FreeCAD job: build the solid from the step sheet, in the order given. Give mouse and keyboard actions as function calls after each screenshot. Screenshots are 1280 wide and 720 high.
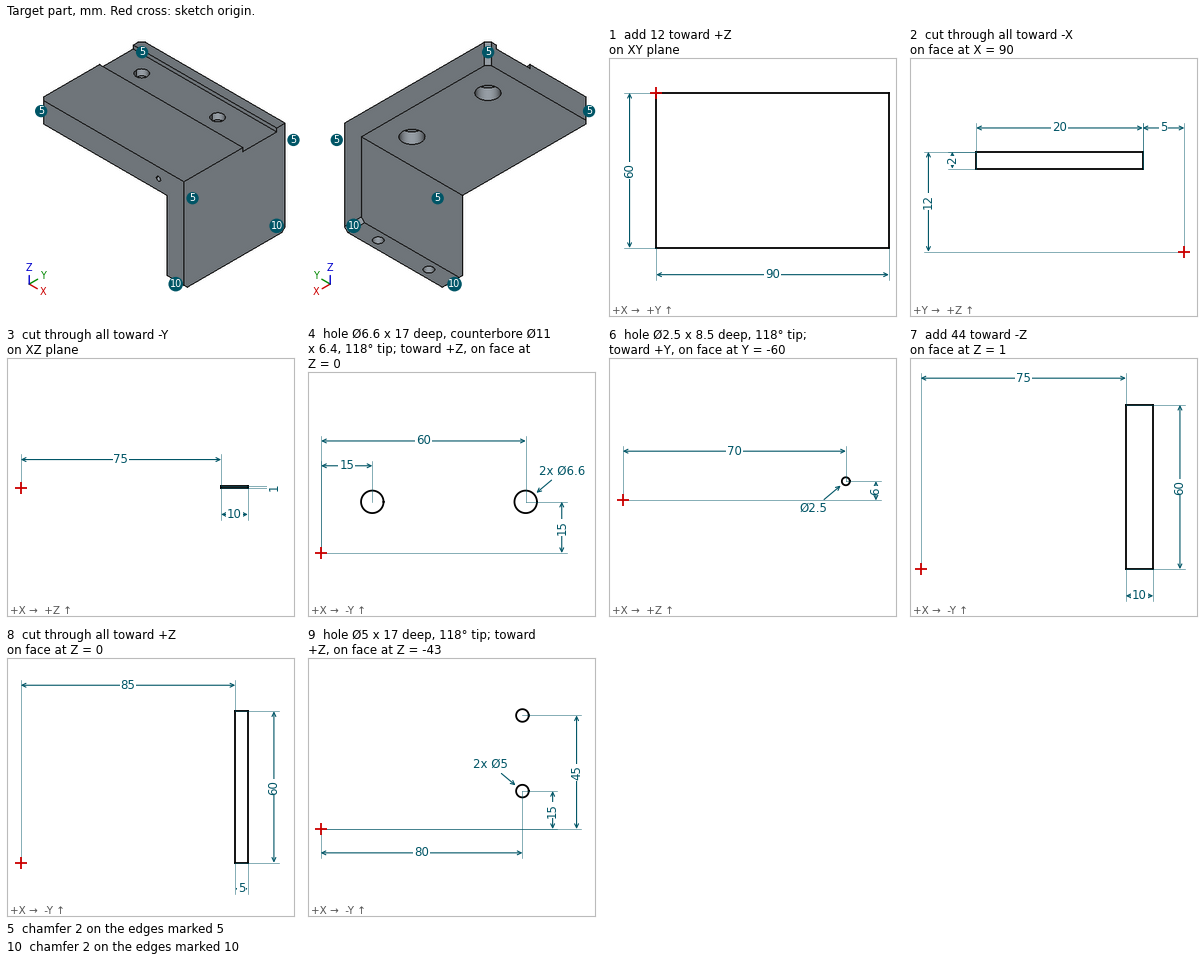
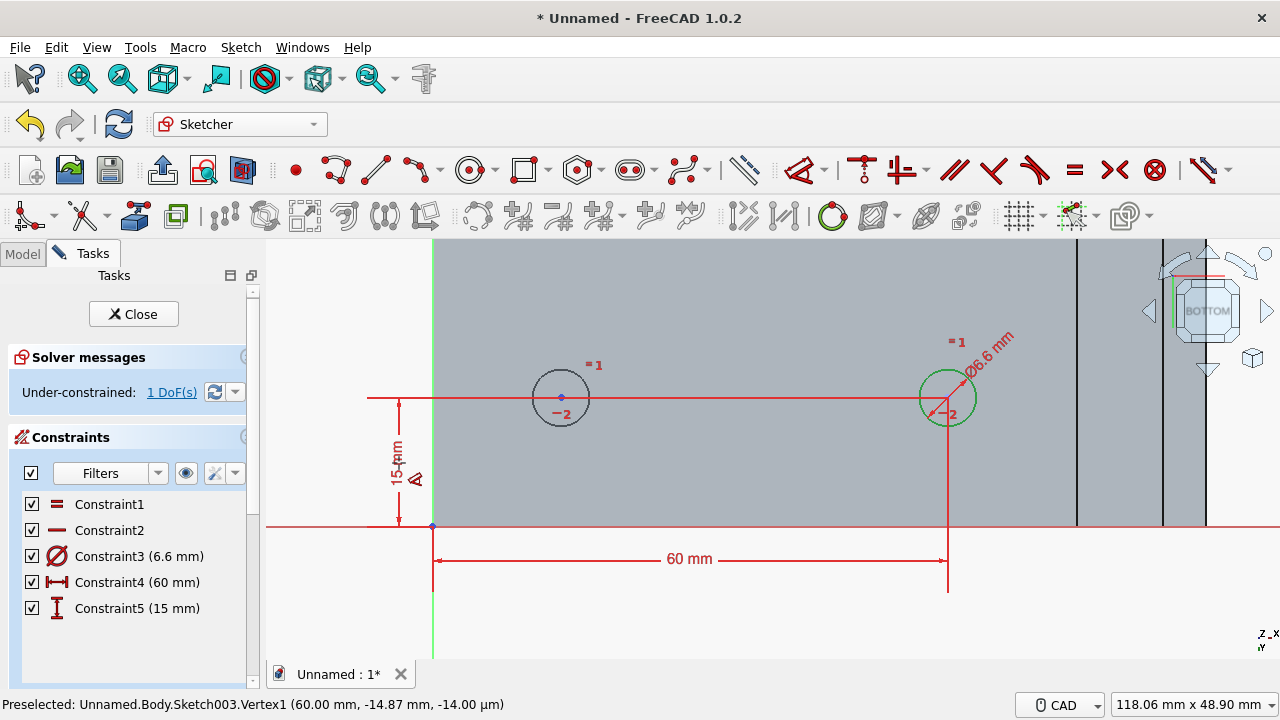
click(561, 398)
click(497, 561)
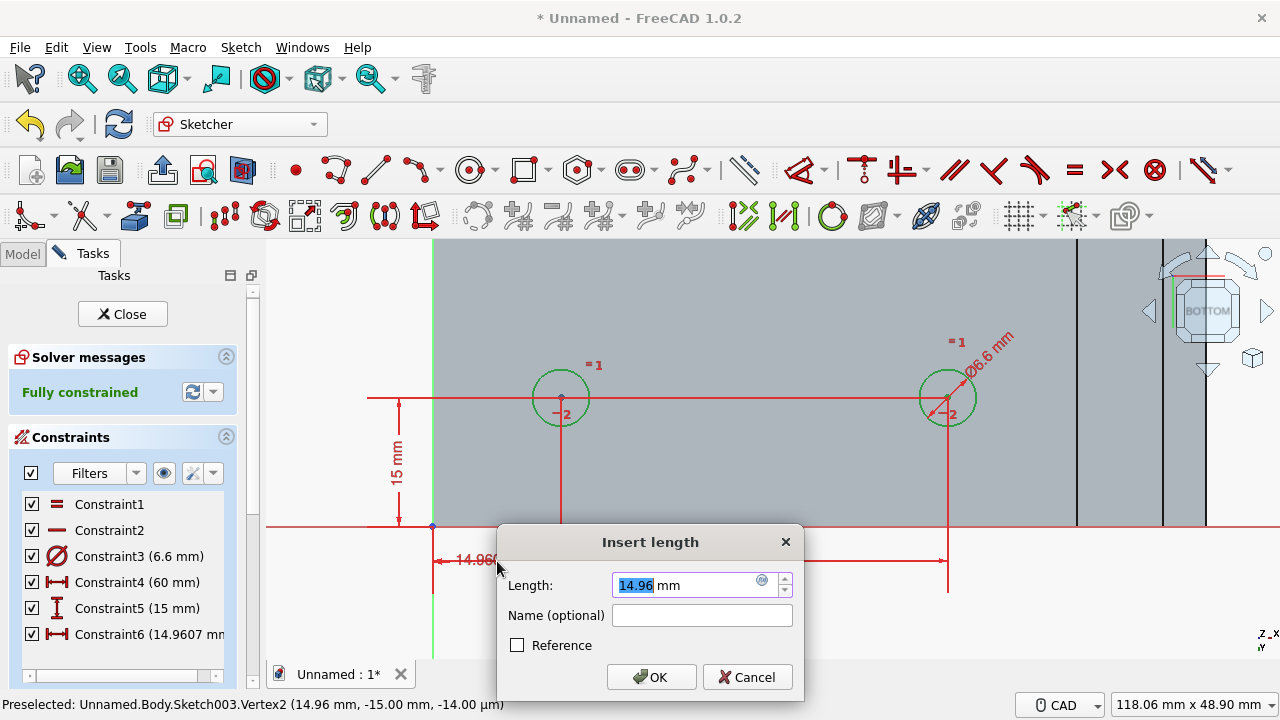
text(15)
key(Return)
key(Escape)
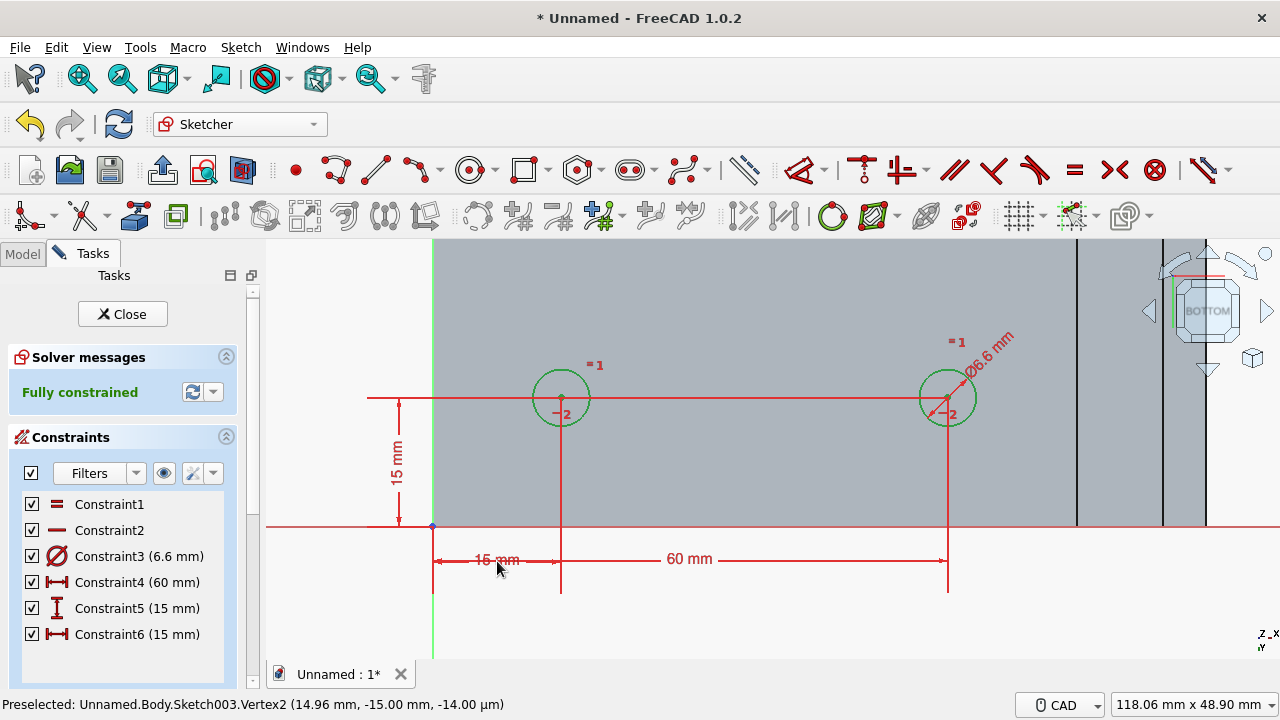
click(123, 314)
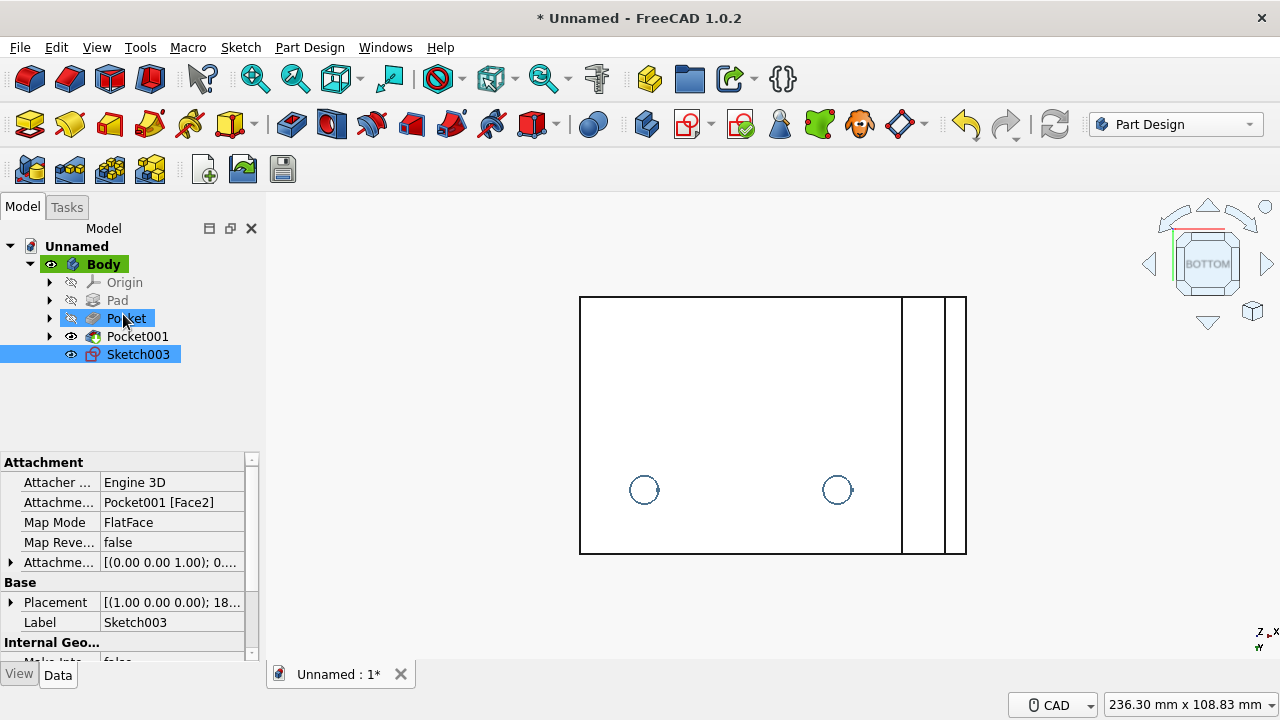
click(332, 124)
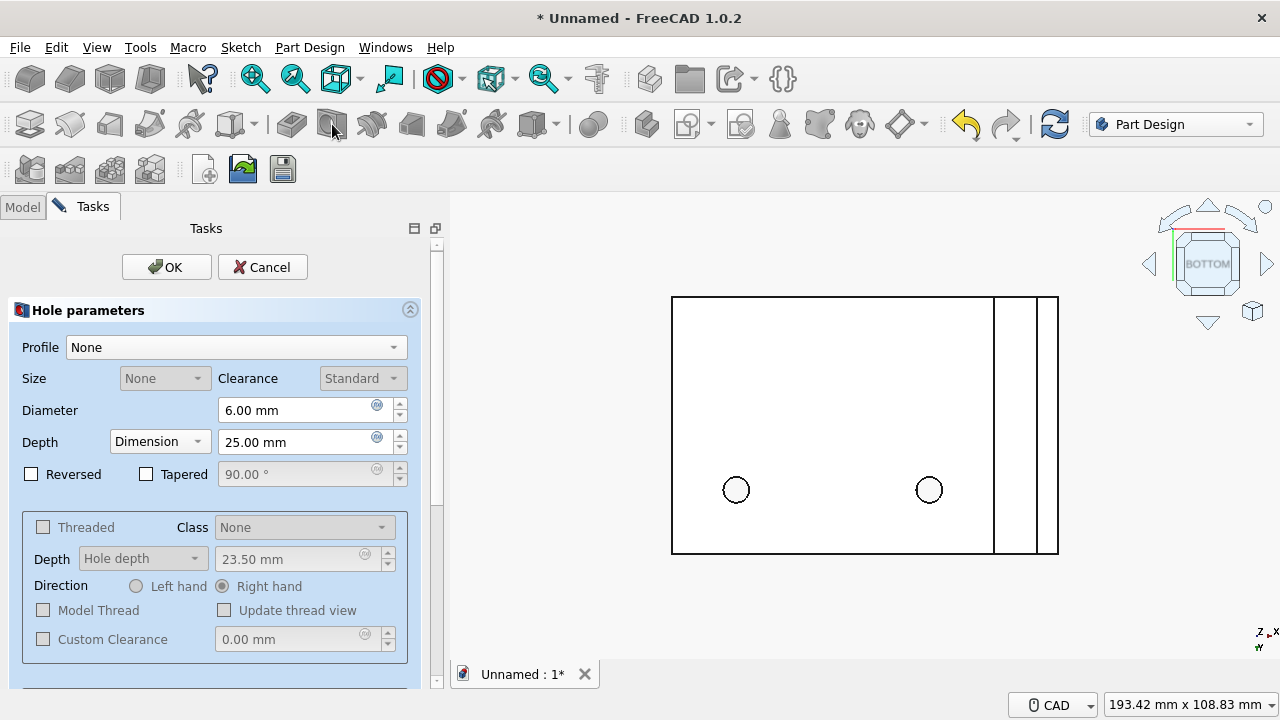
triple_click(305, 410)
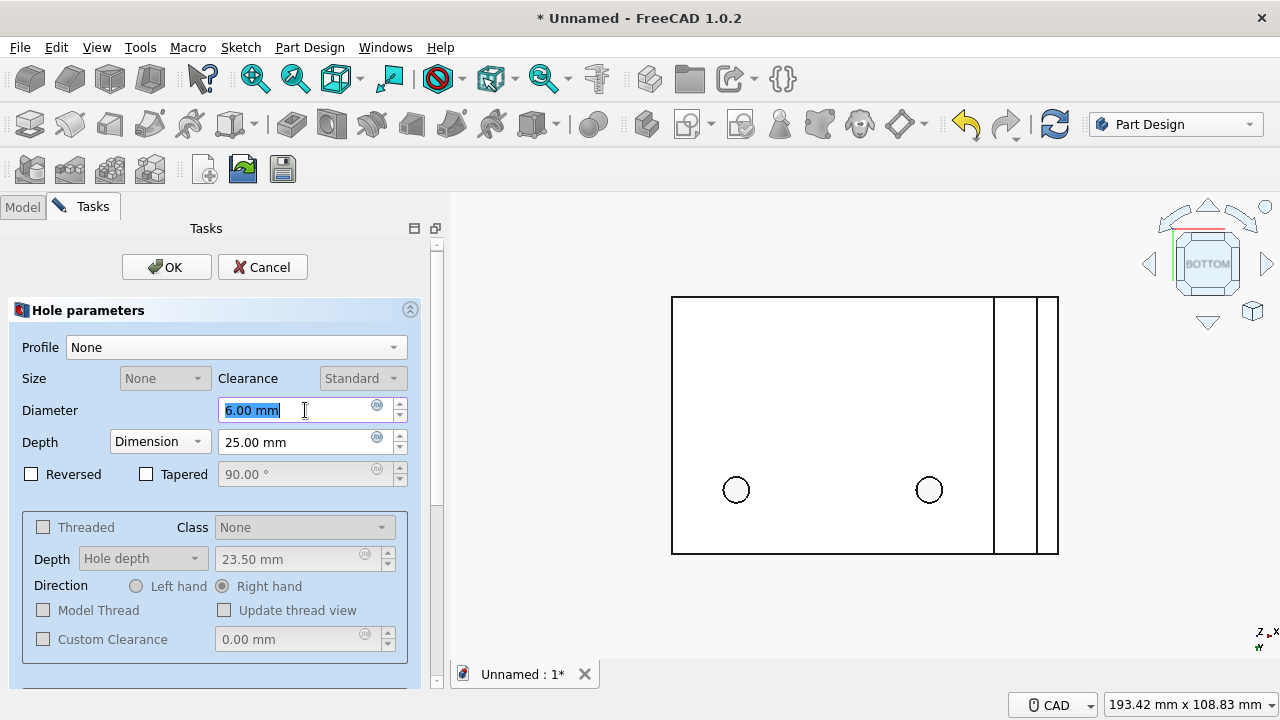
text(6.6)
key(Tab)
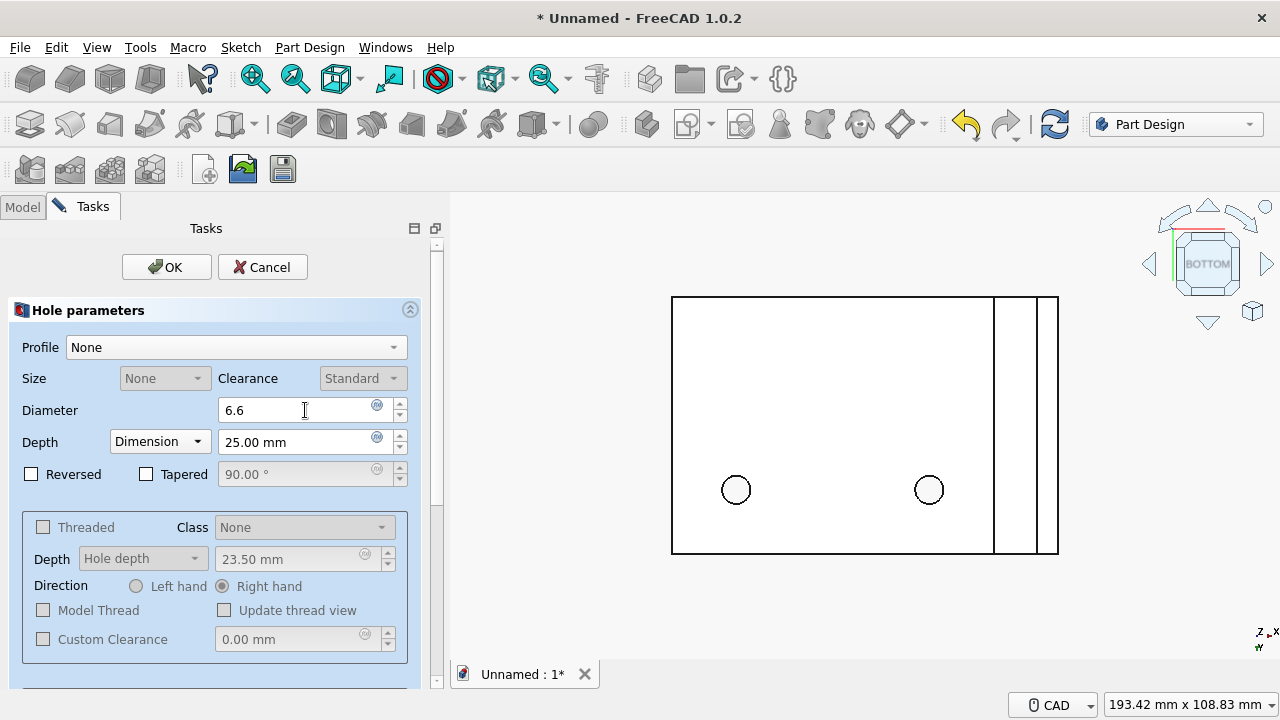
triple_click(305, 442)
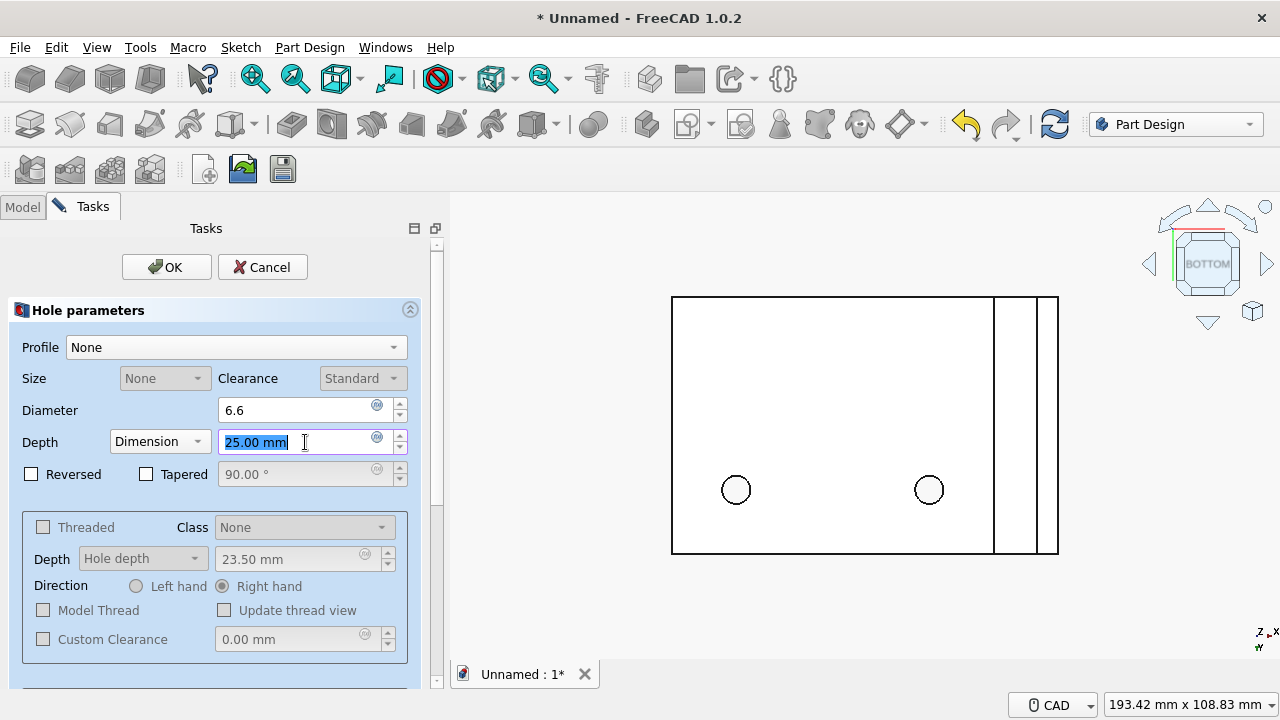
text(17)
key(Tab)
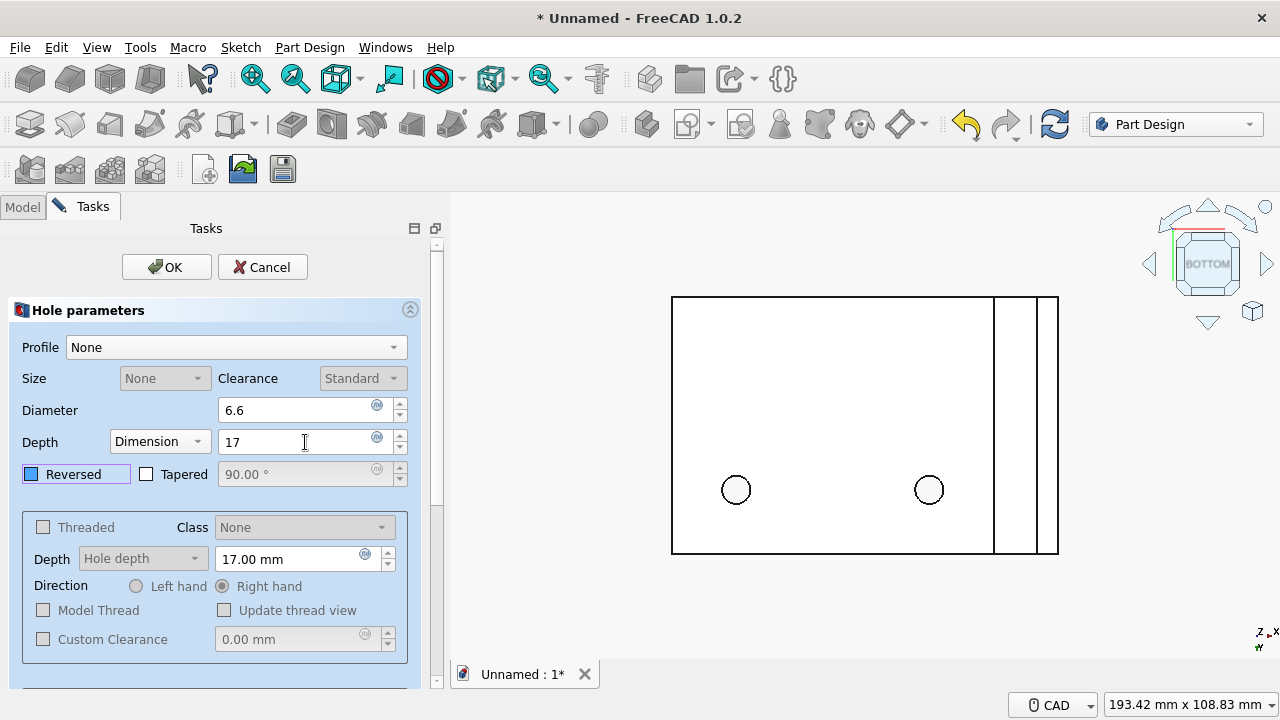
scroll(437, 463, down, 2)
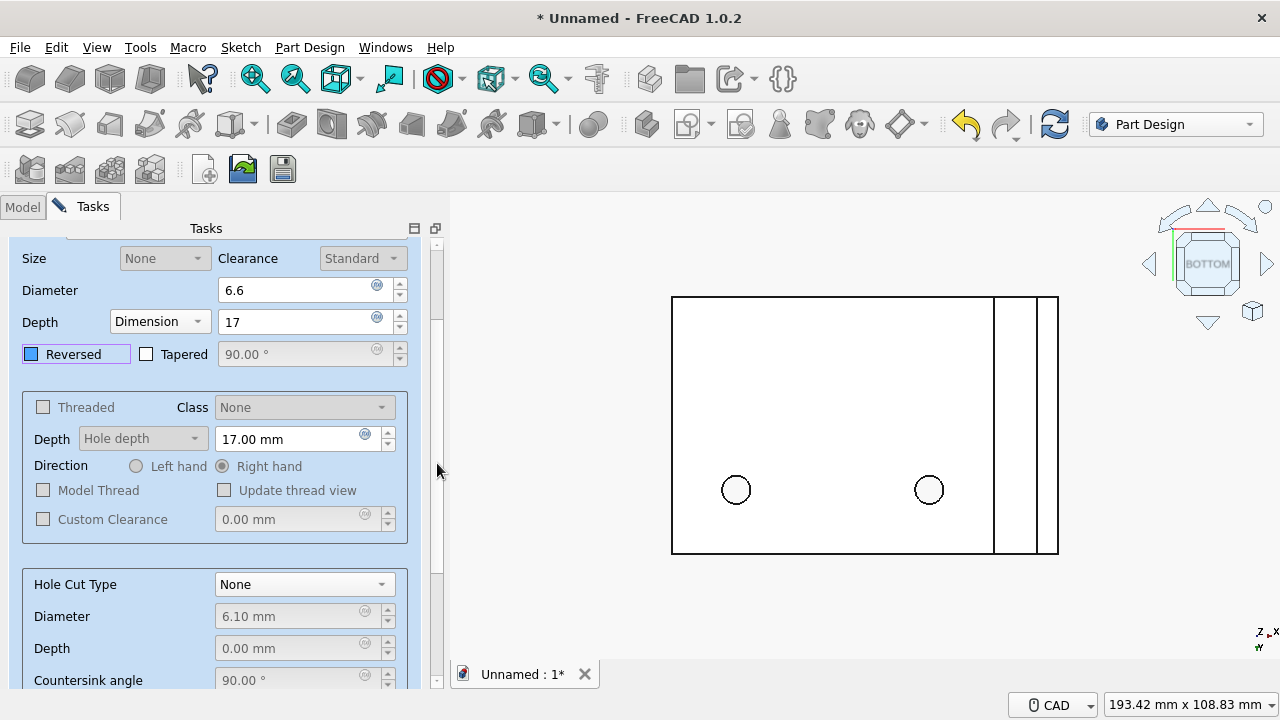
click(306, 584)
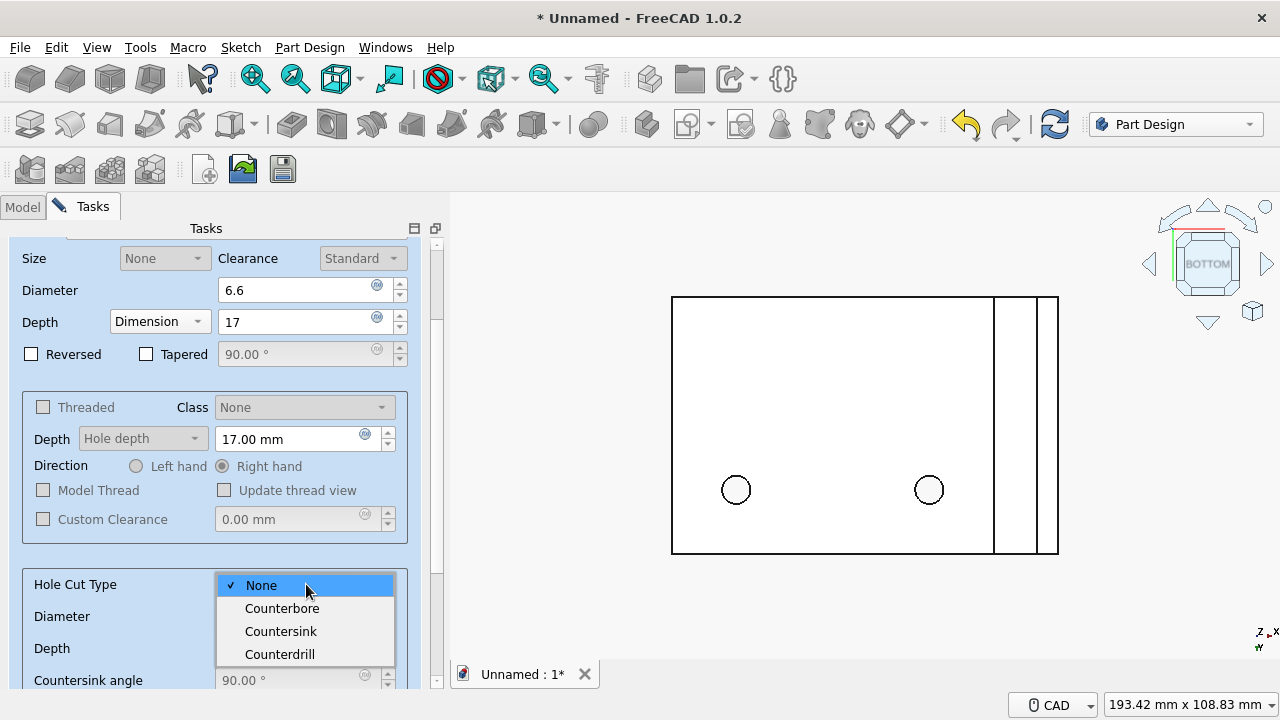
click(304, 608)